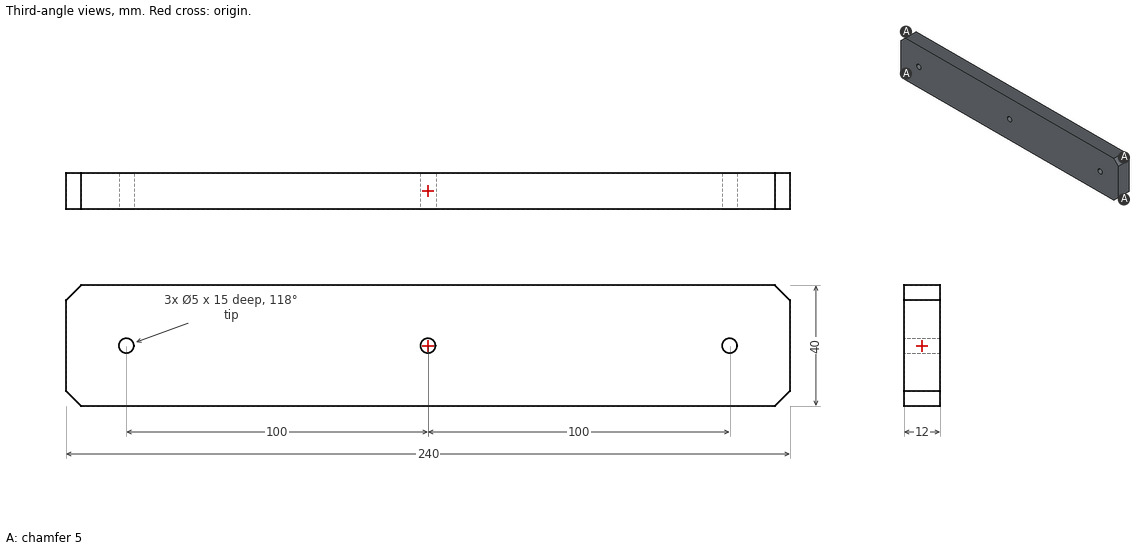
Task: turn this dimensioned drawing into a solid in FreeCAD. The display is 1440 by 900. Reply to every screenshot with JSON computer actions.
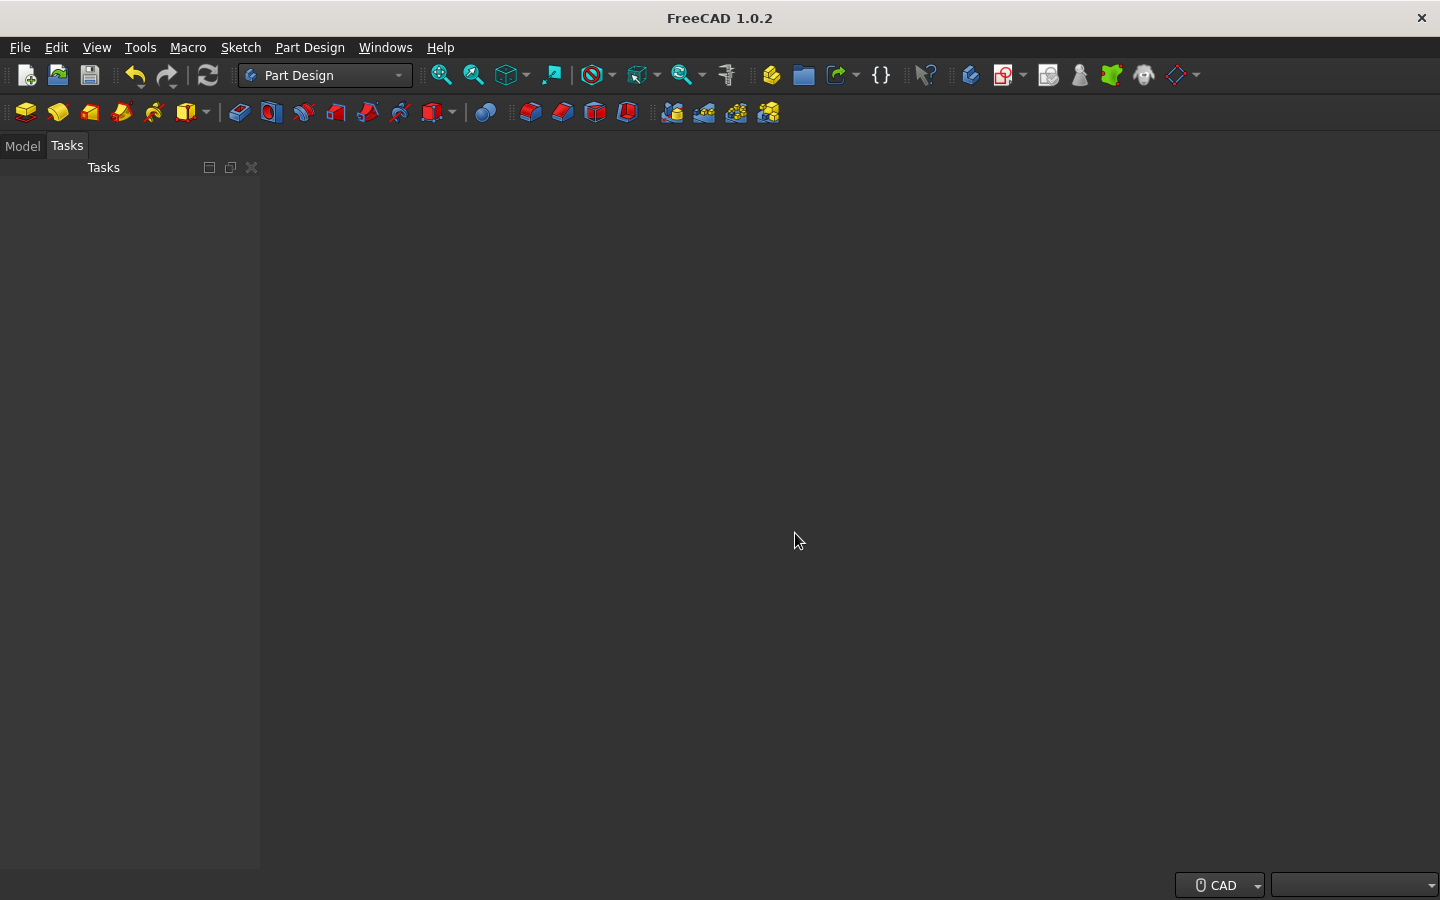
{"action": "left_click", "coordinate": [26, 76]}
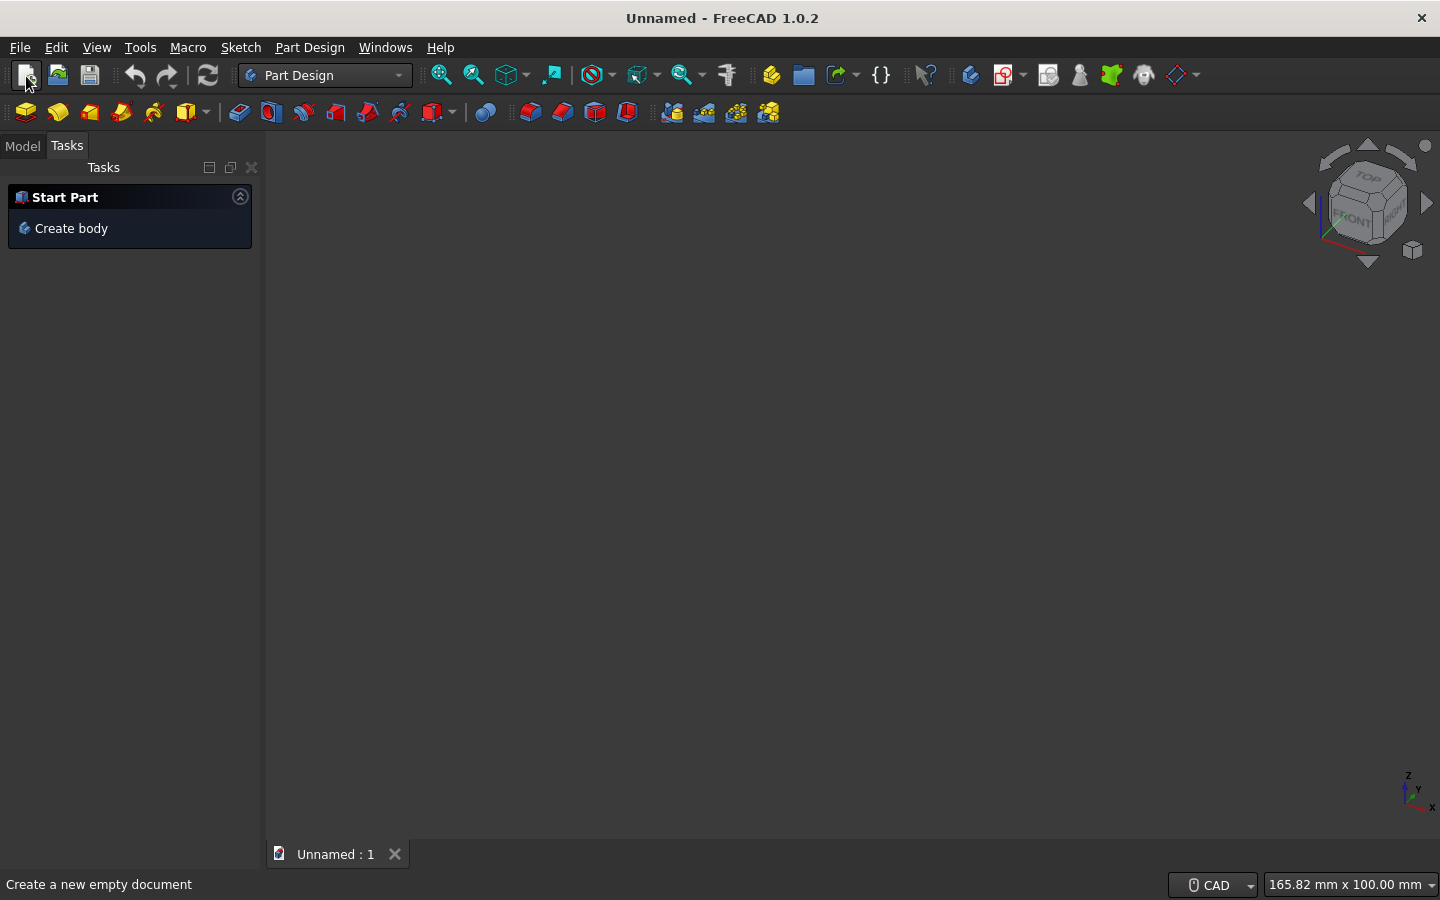
{"action": "left_click", "coordinate": [1004, 76]}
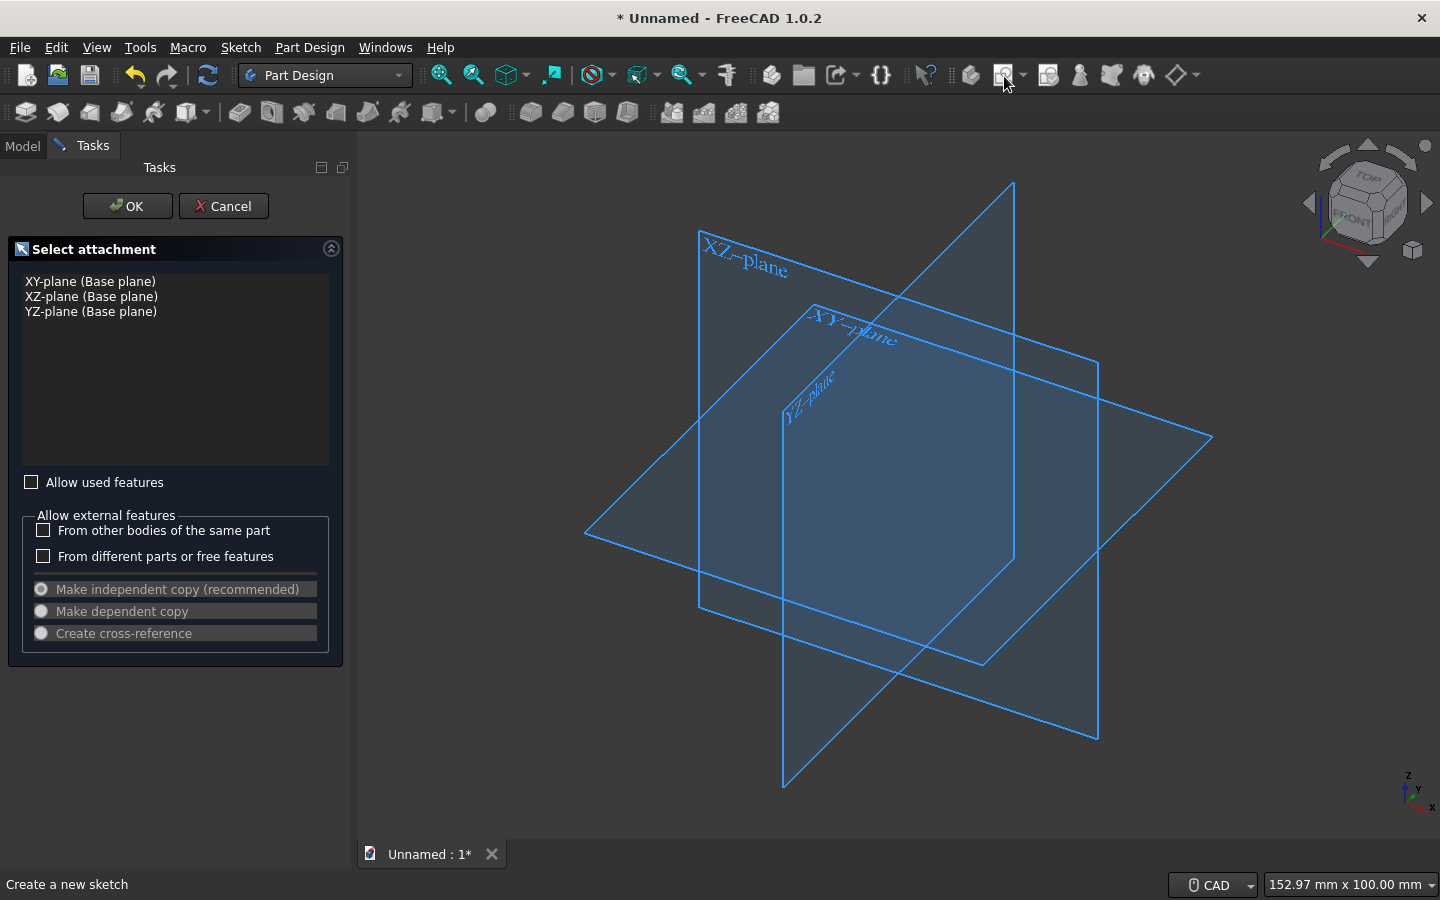
{"action": "left_click", "coordinate": [82, 296]}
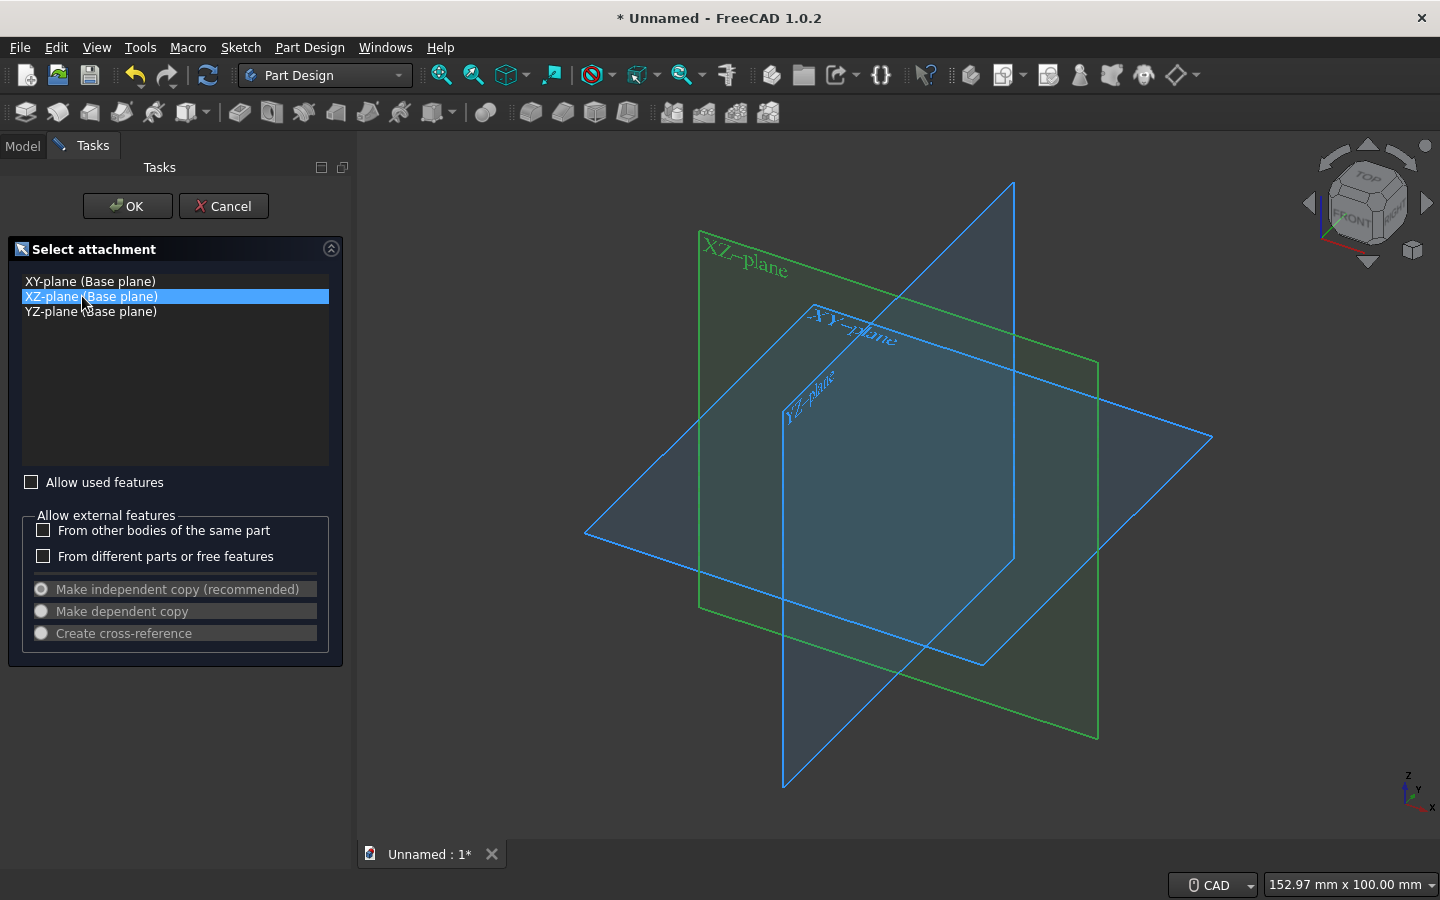
{"action": "left_click", "coordinate": [128, 206]}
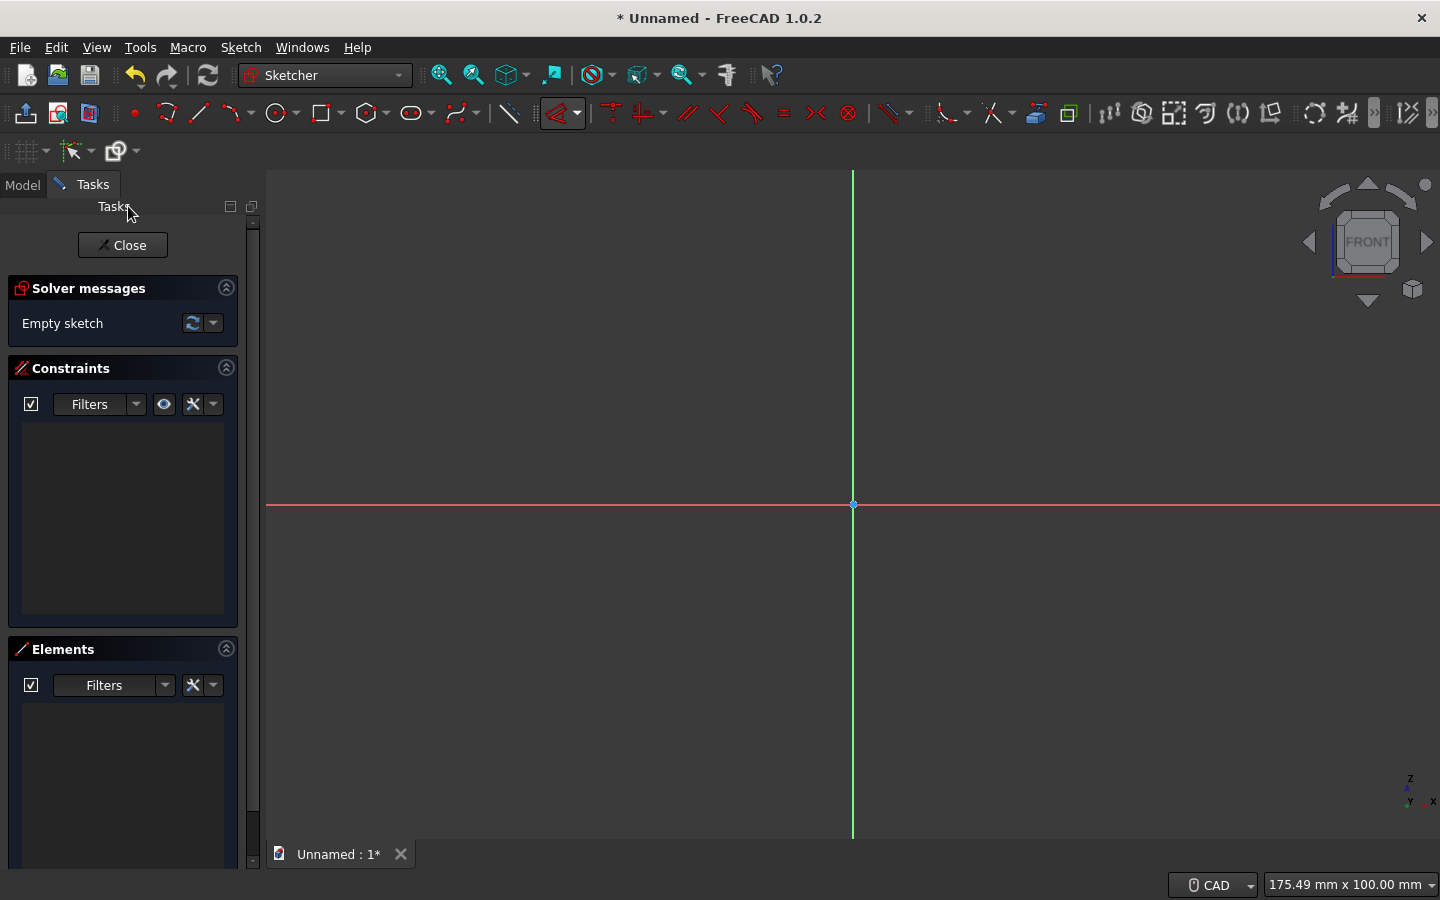
{"action": "scroll", "coordinate": [729, 505], "scroll_direction": "down", "scroll_amount": 4}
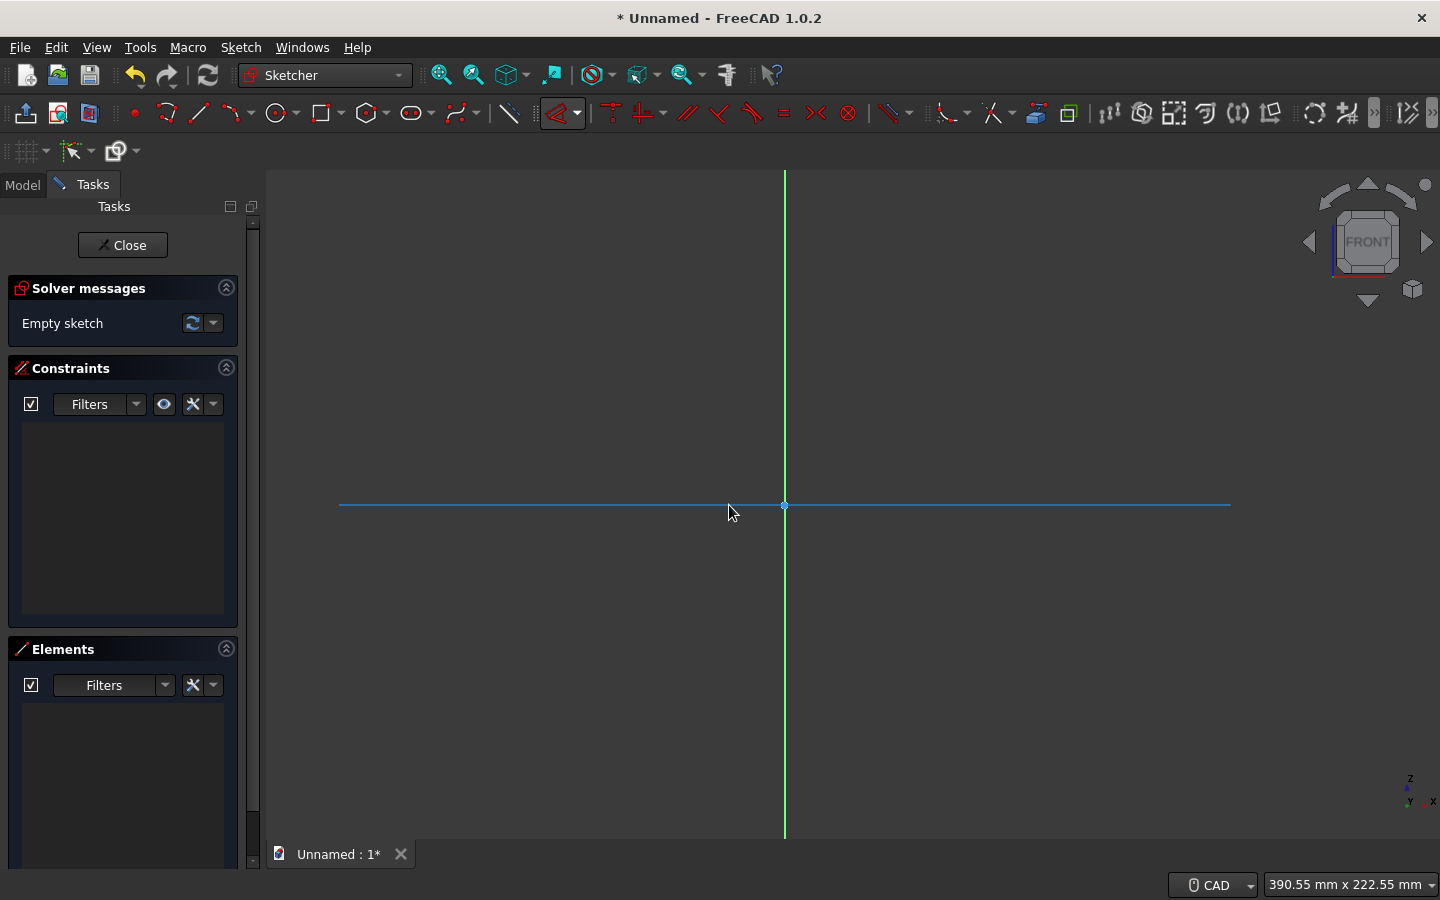
{"action": "key", "text": "g v"}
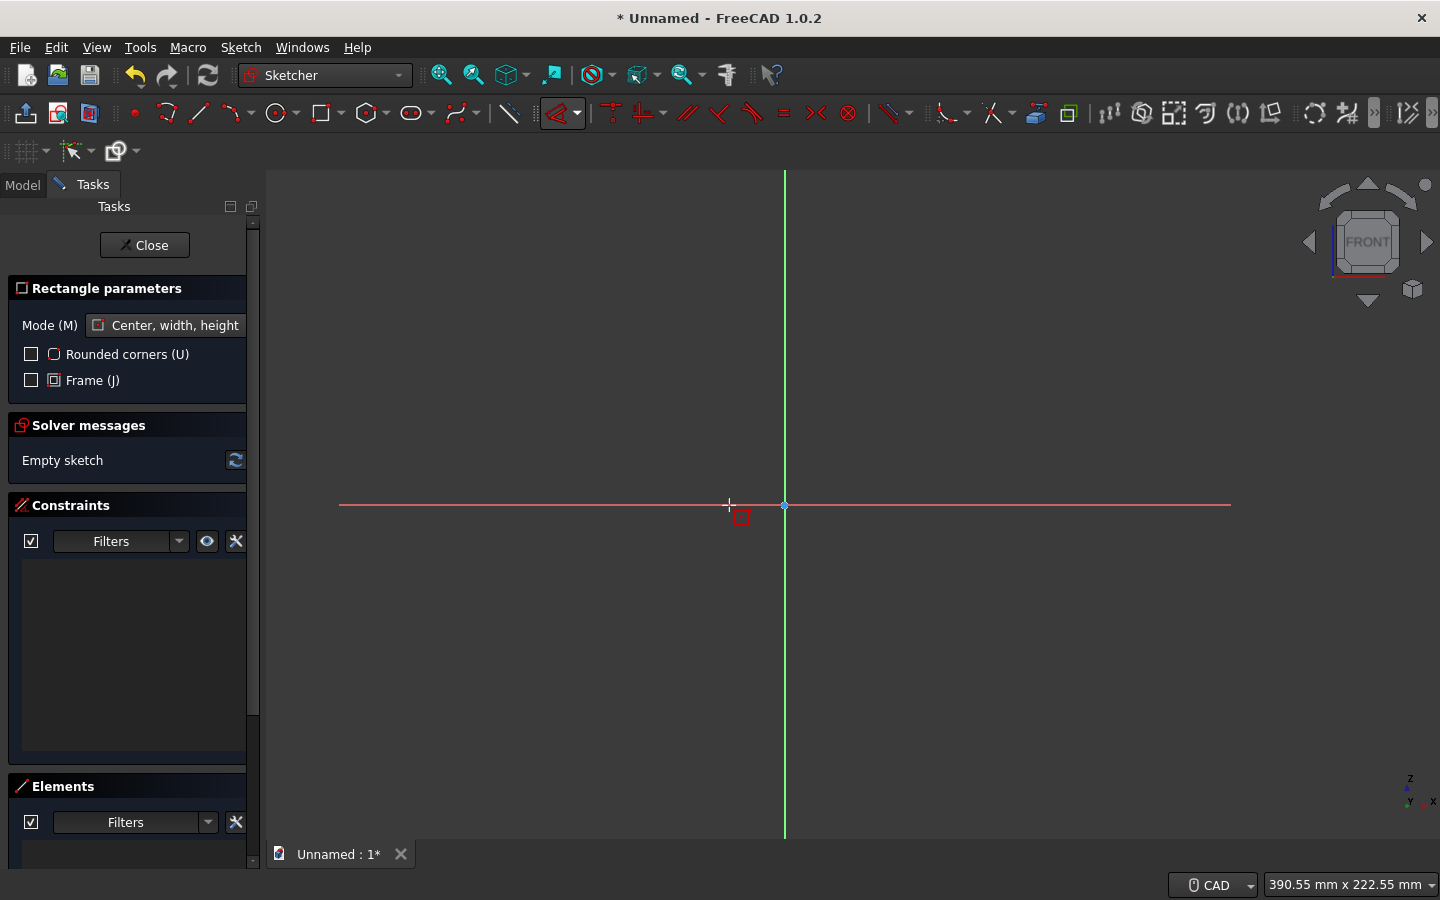
{"action": "left_click", "coordinate": [785, 505]}
{"action": "left_click", "coordinate": [1146, 445]}
{"action": "key", "text": "Escape"}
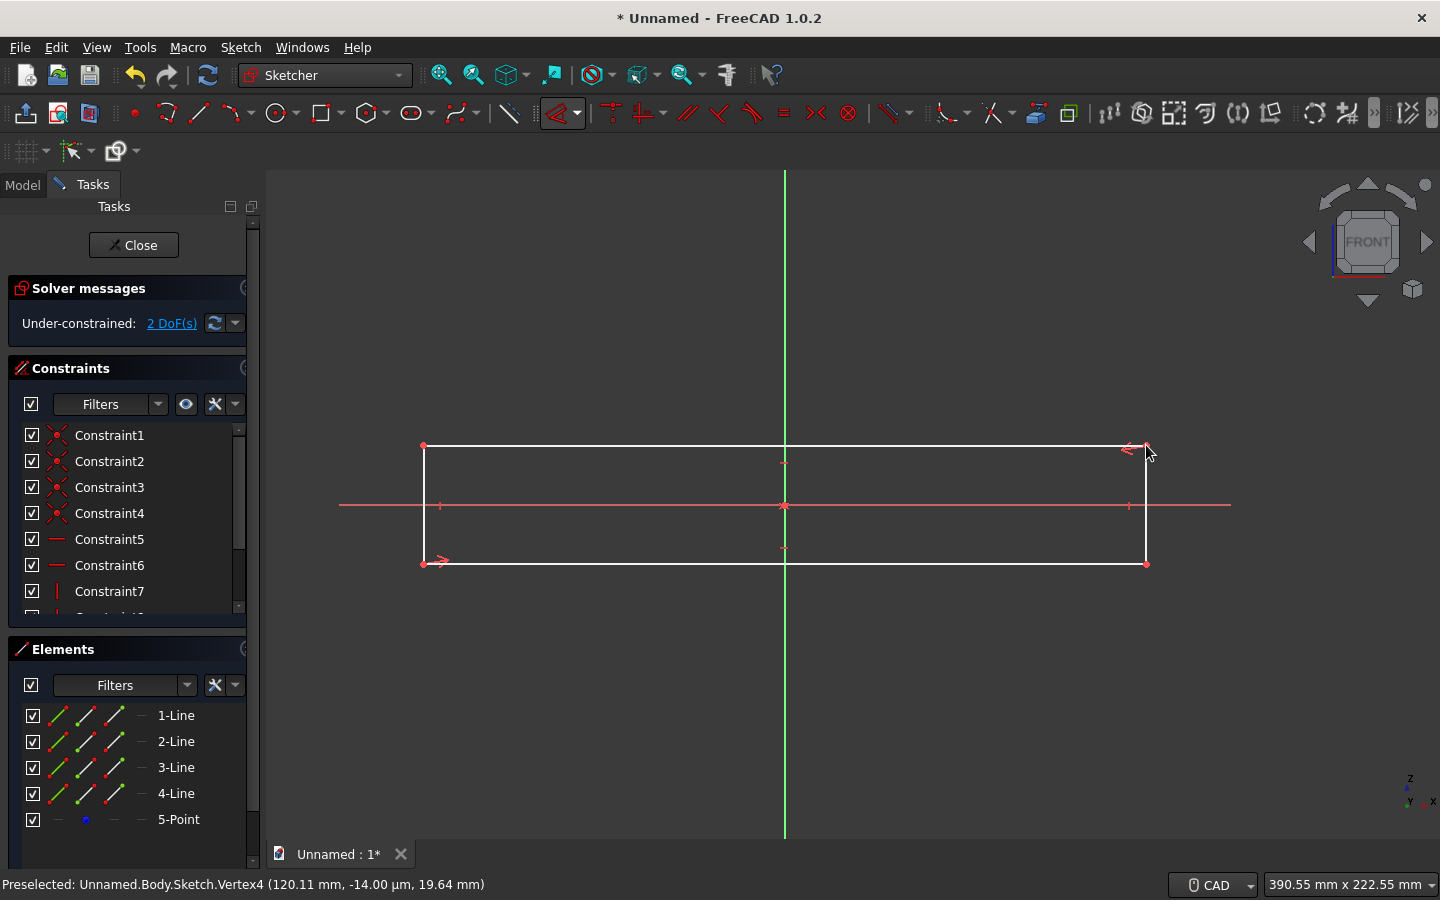
{"action": "left_click", "coordinate": [1146, 529]}